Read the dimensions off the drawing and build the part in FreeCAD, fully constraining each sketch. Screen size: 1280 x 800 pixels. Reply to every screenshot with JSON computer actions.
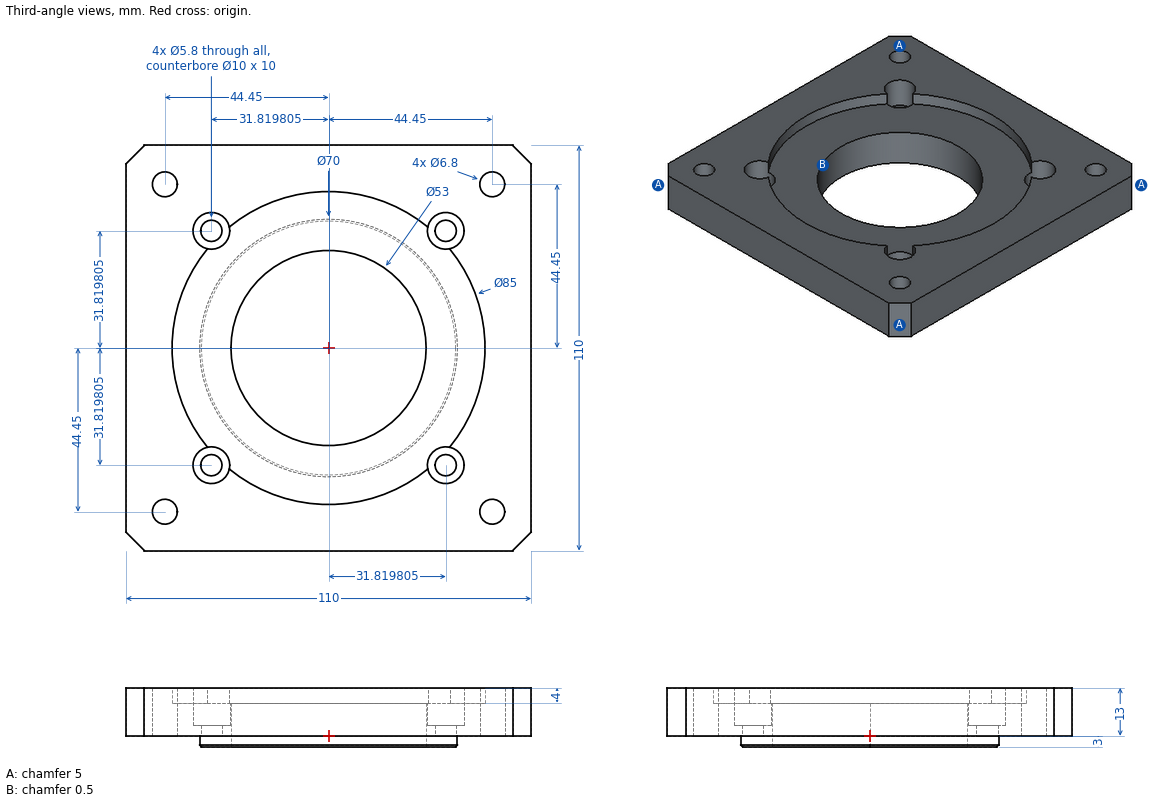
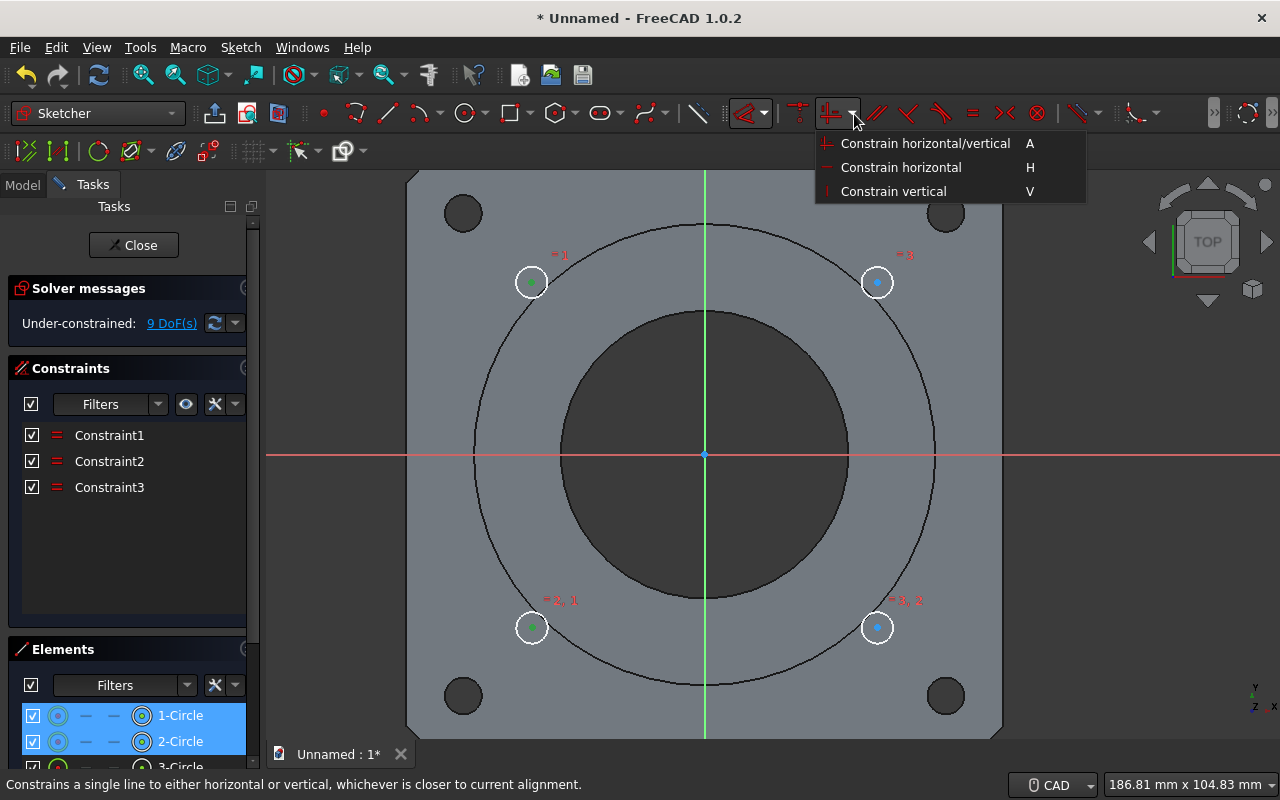
{"action": "left_click", "coordinate": [951, 191]}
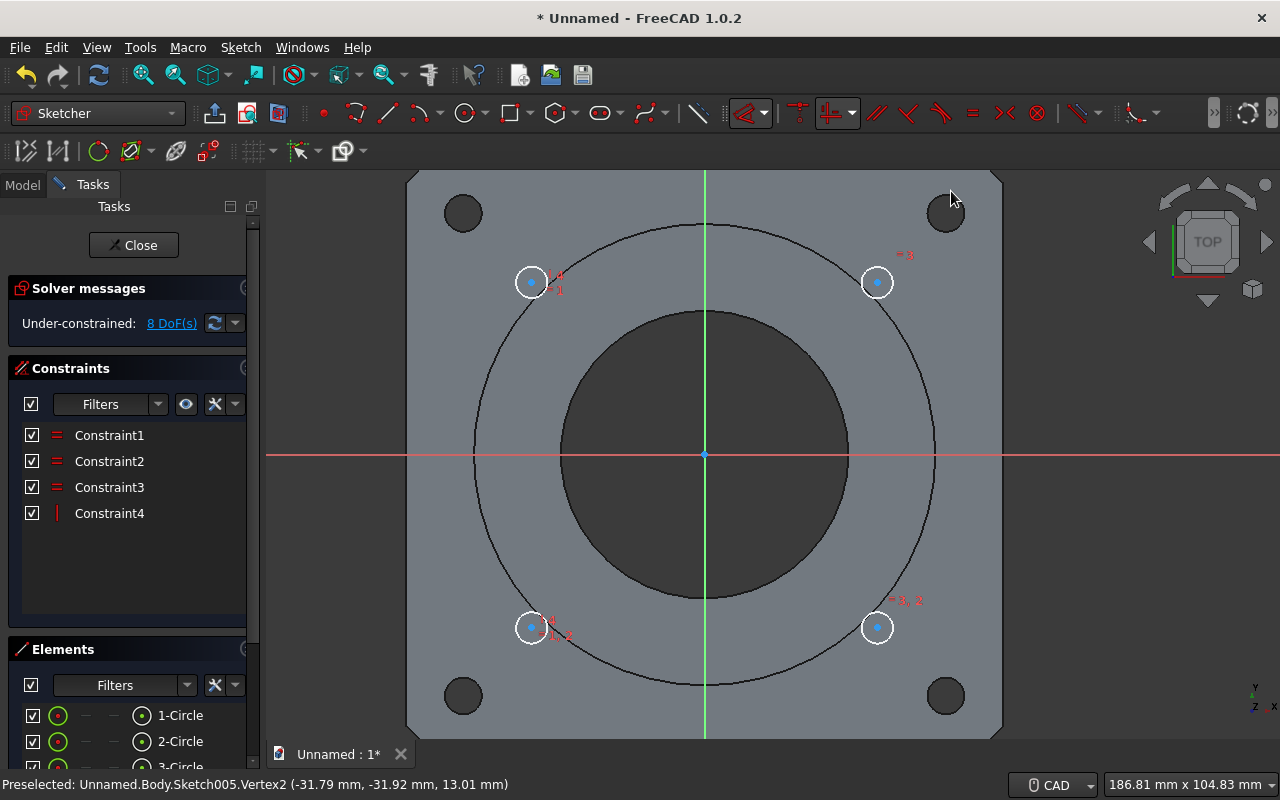
{"action": "left_click", "coordinate": [532, 628]}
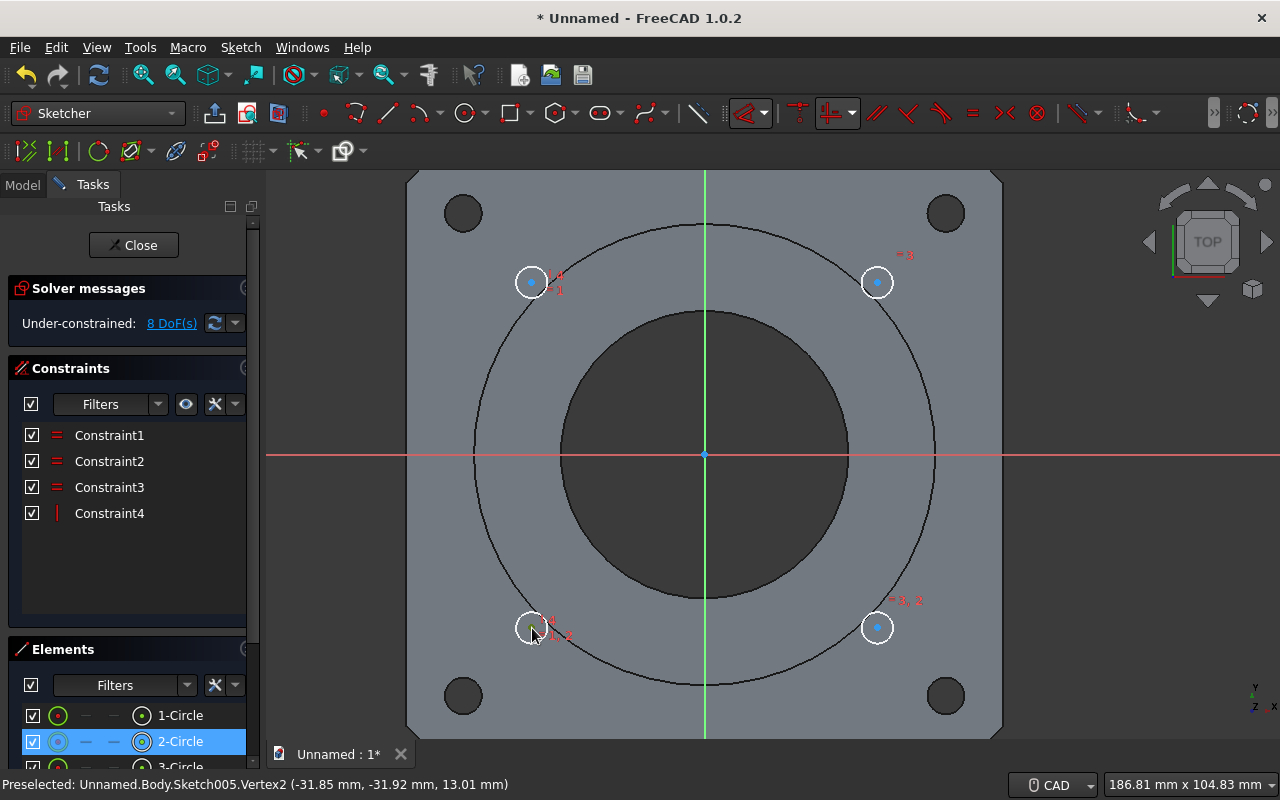
{"action": "left_click", "coordinate": [877, 628]}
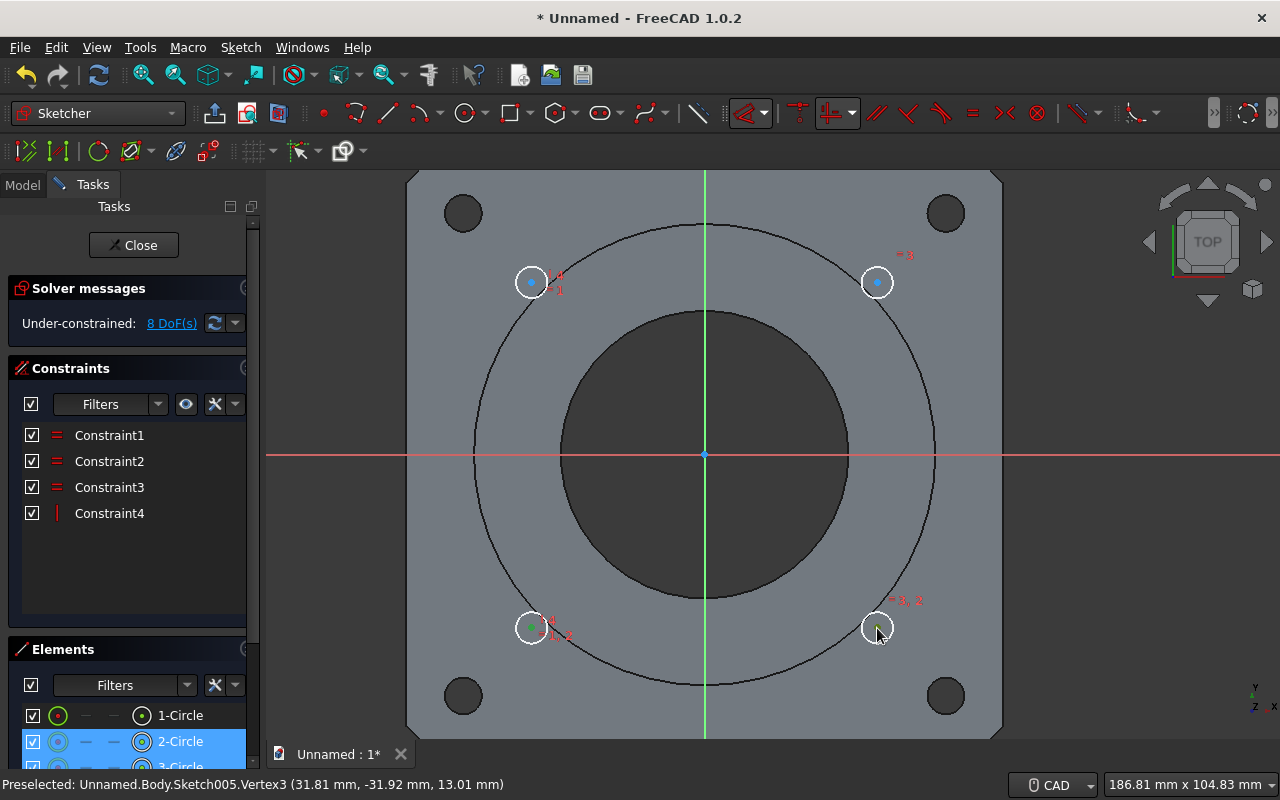
{"action": "key", "text": "h"}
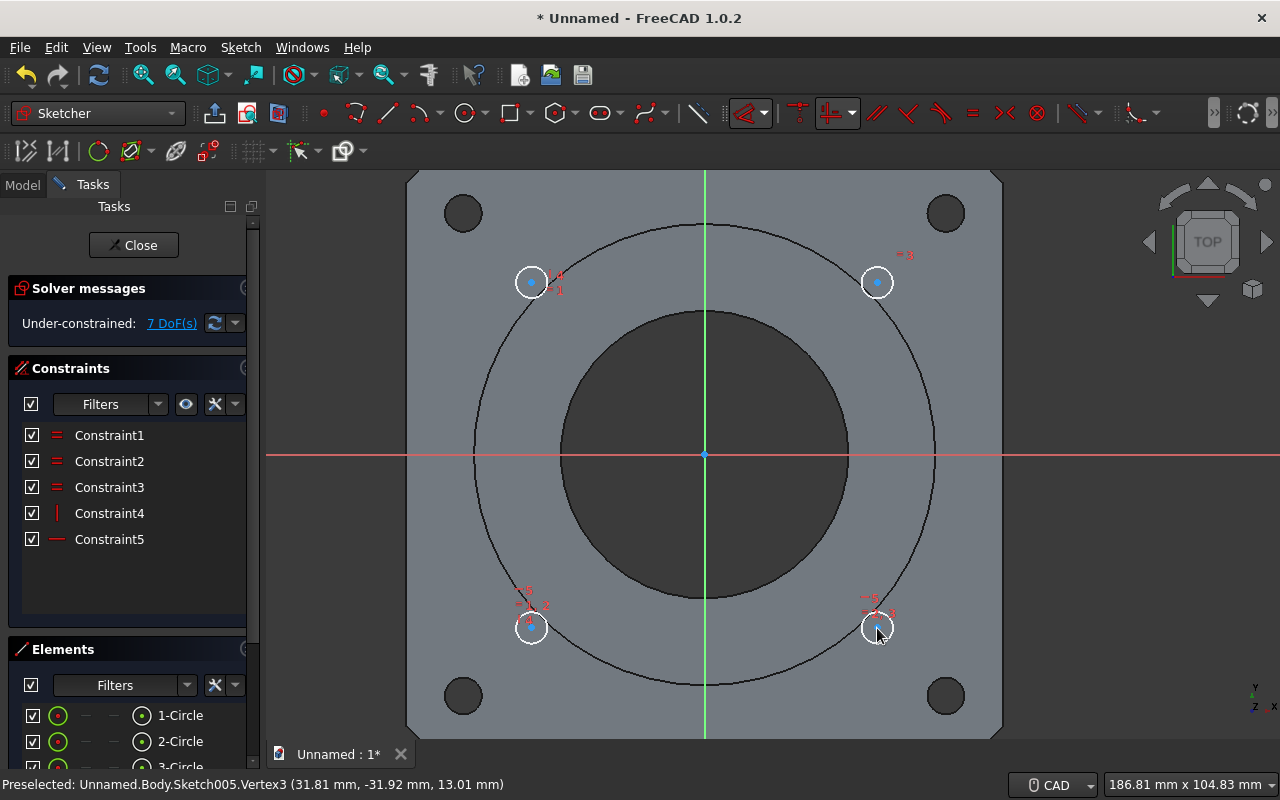
{"action": "left_click", "coordinate": [877, 628]}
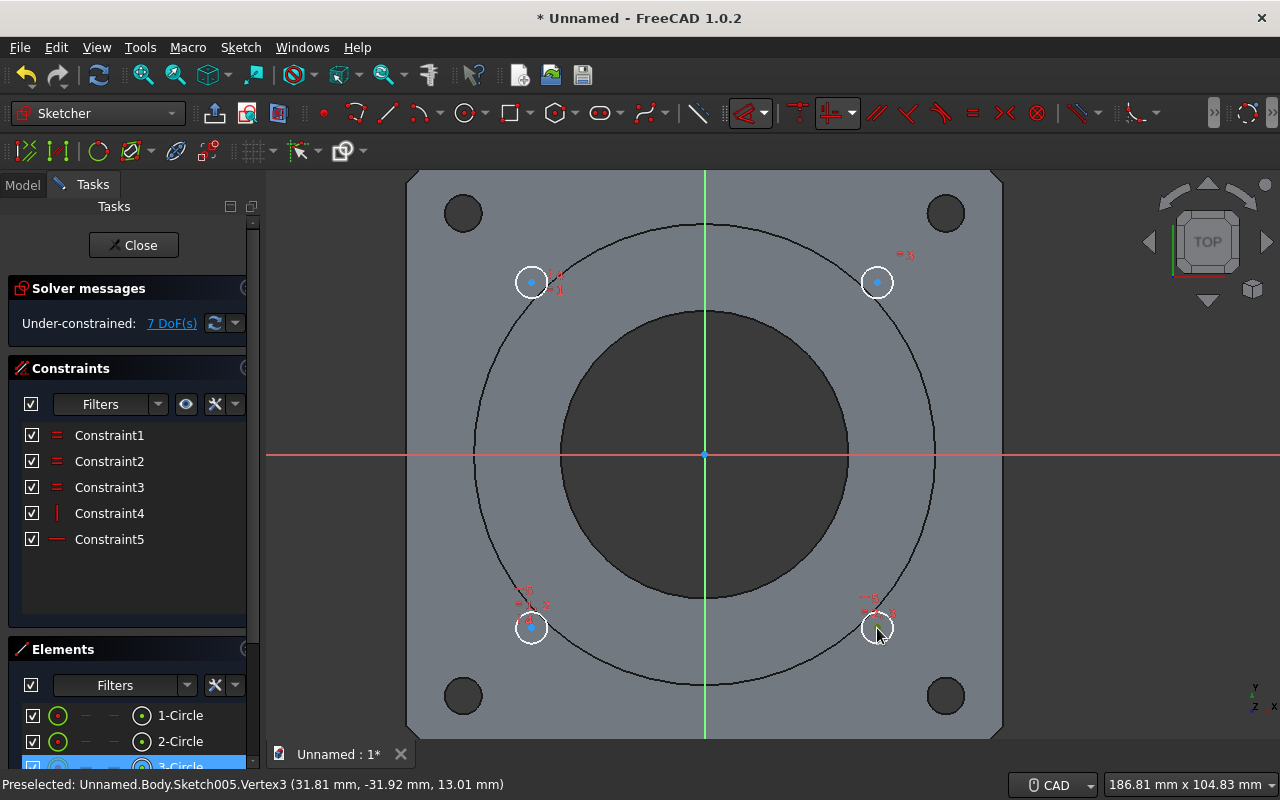
{"action": "left_click", "coordinate": [877, 283]}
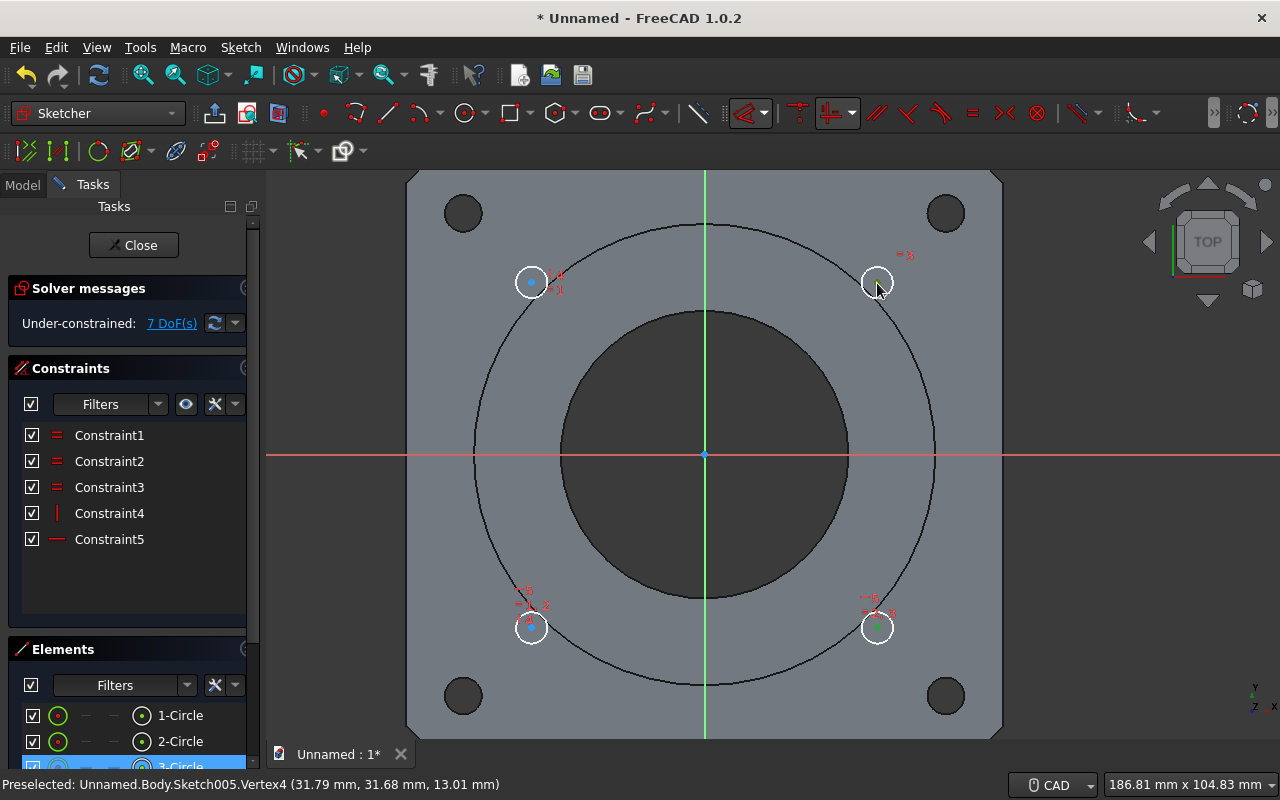
{"action": "key", "text": "v"}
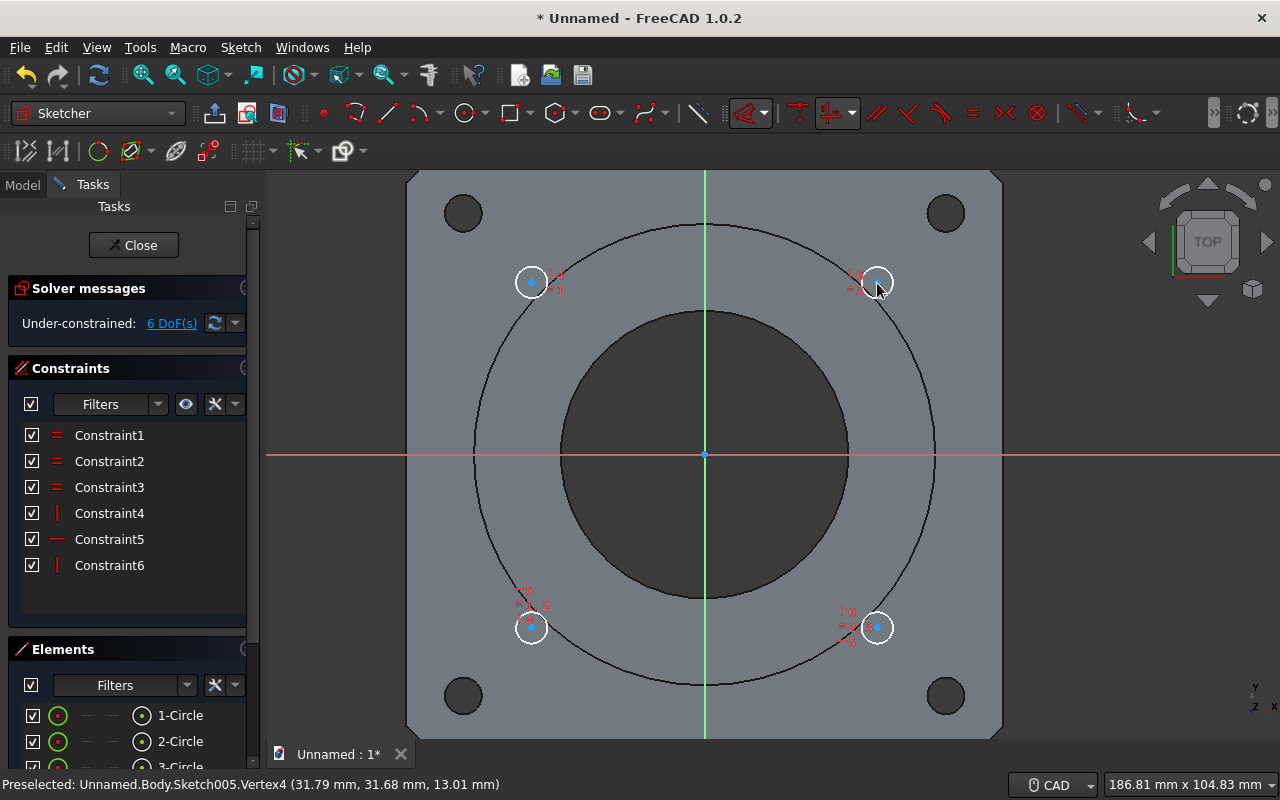
{"action": "left_click", "coordinate": [532, 282]}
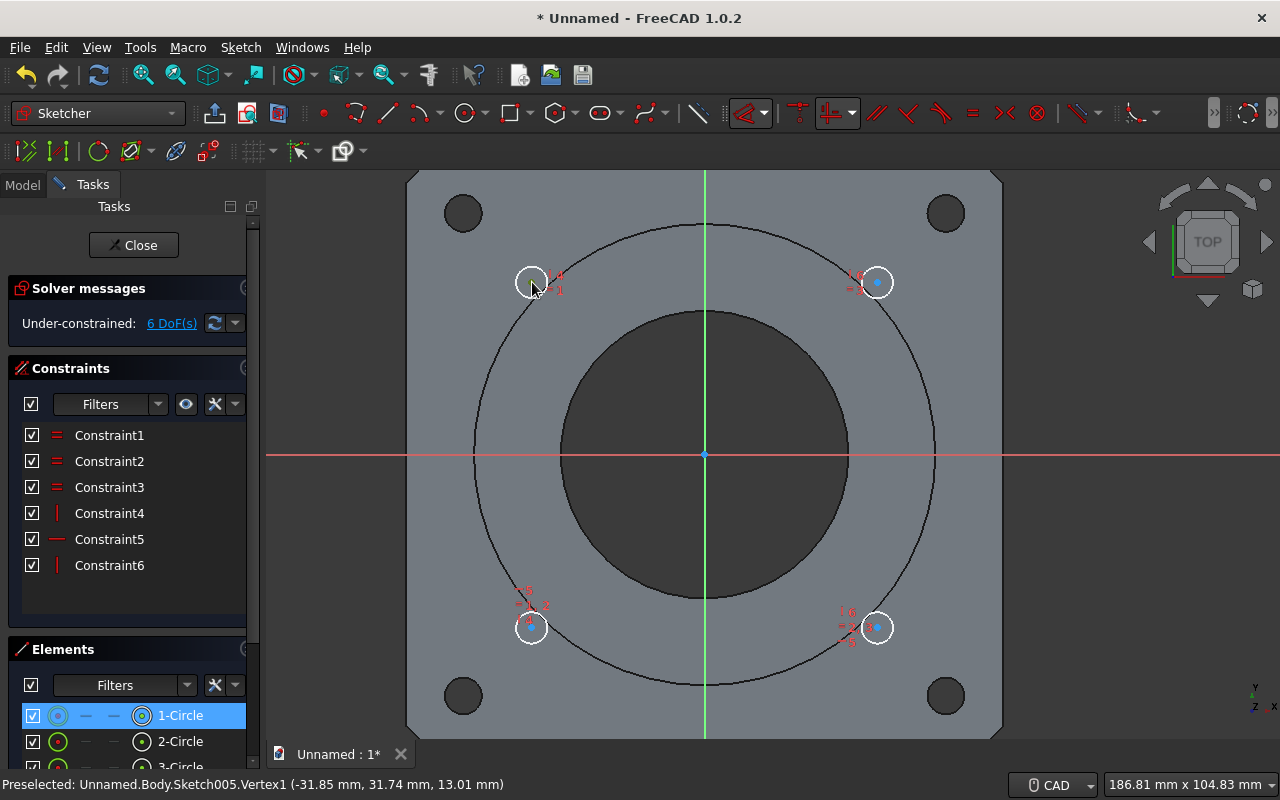
{"action": "left_click", "coordinate": [877, 283]}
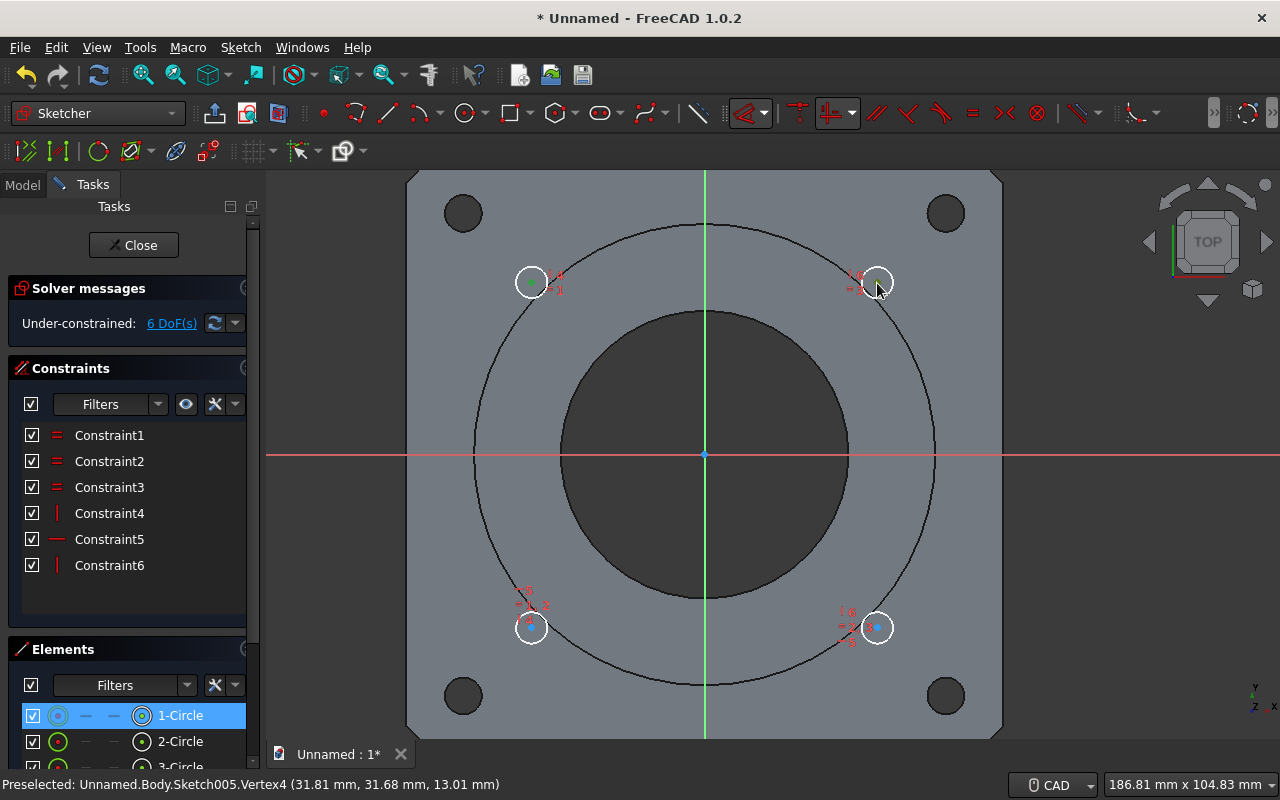
{"action": "key", "text": "h"}